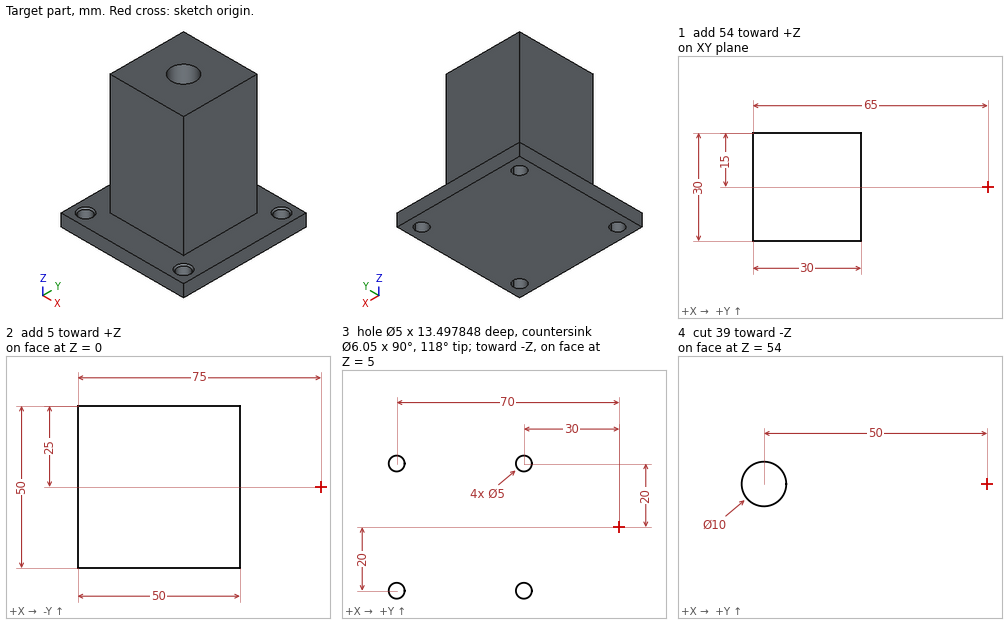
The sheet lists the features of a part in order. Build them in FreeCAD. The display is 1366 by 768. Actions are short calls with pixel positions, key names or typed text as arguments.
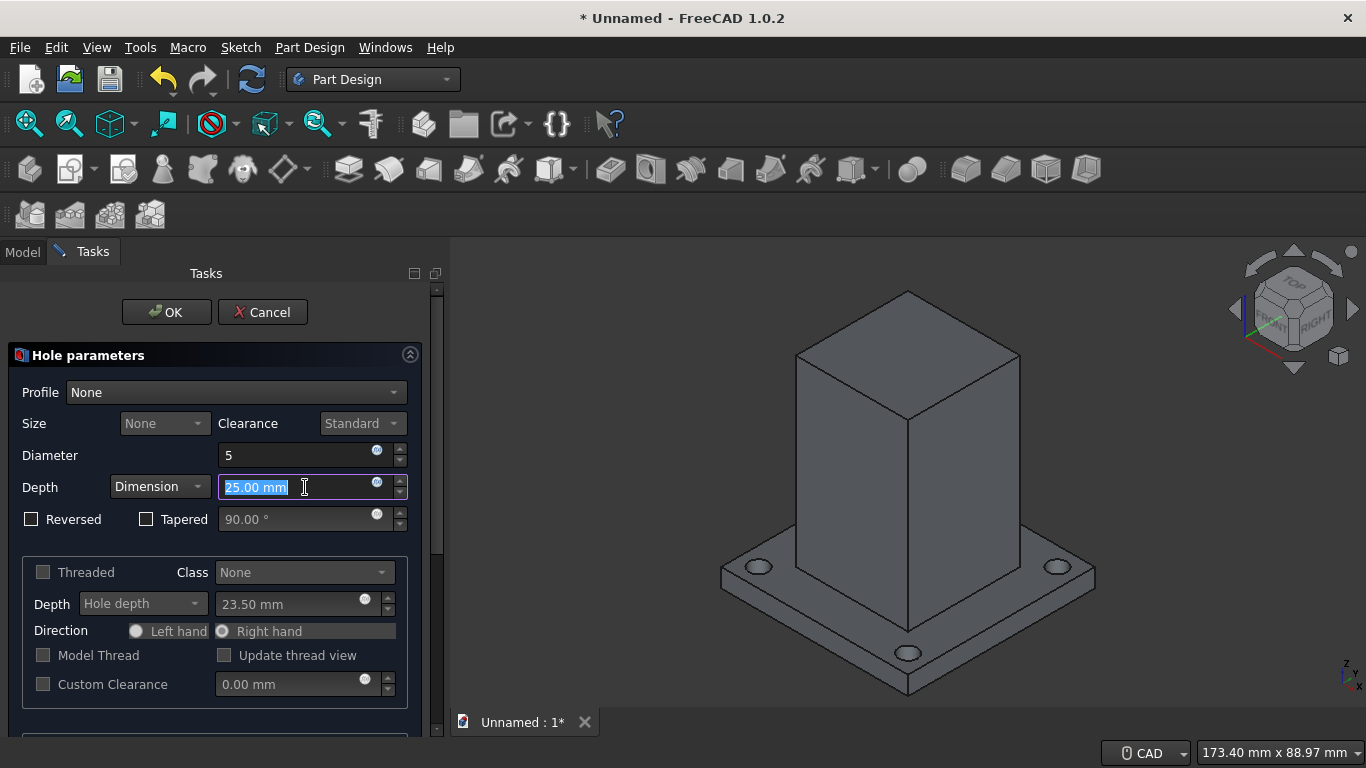
text(13.497848)
key(Tab)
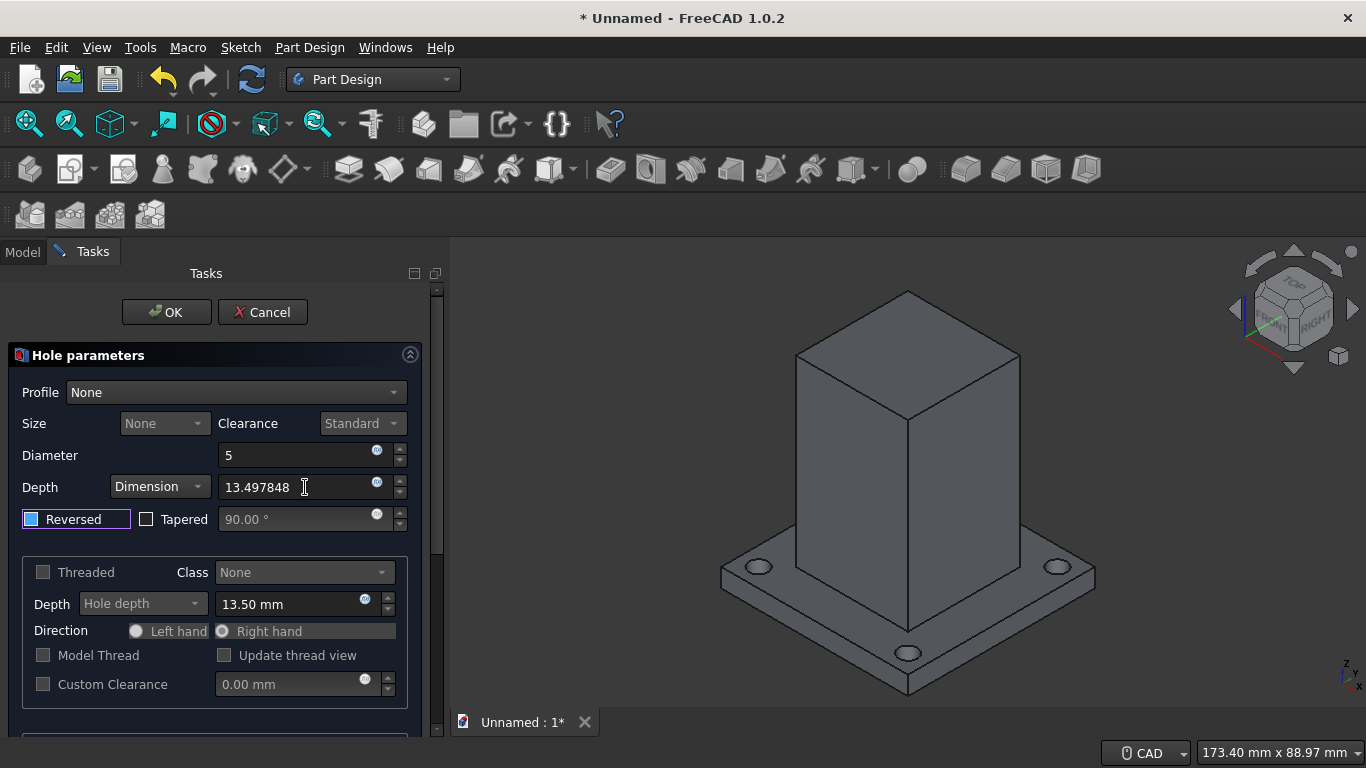
scroll(437, 510, down, 2)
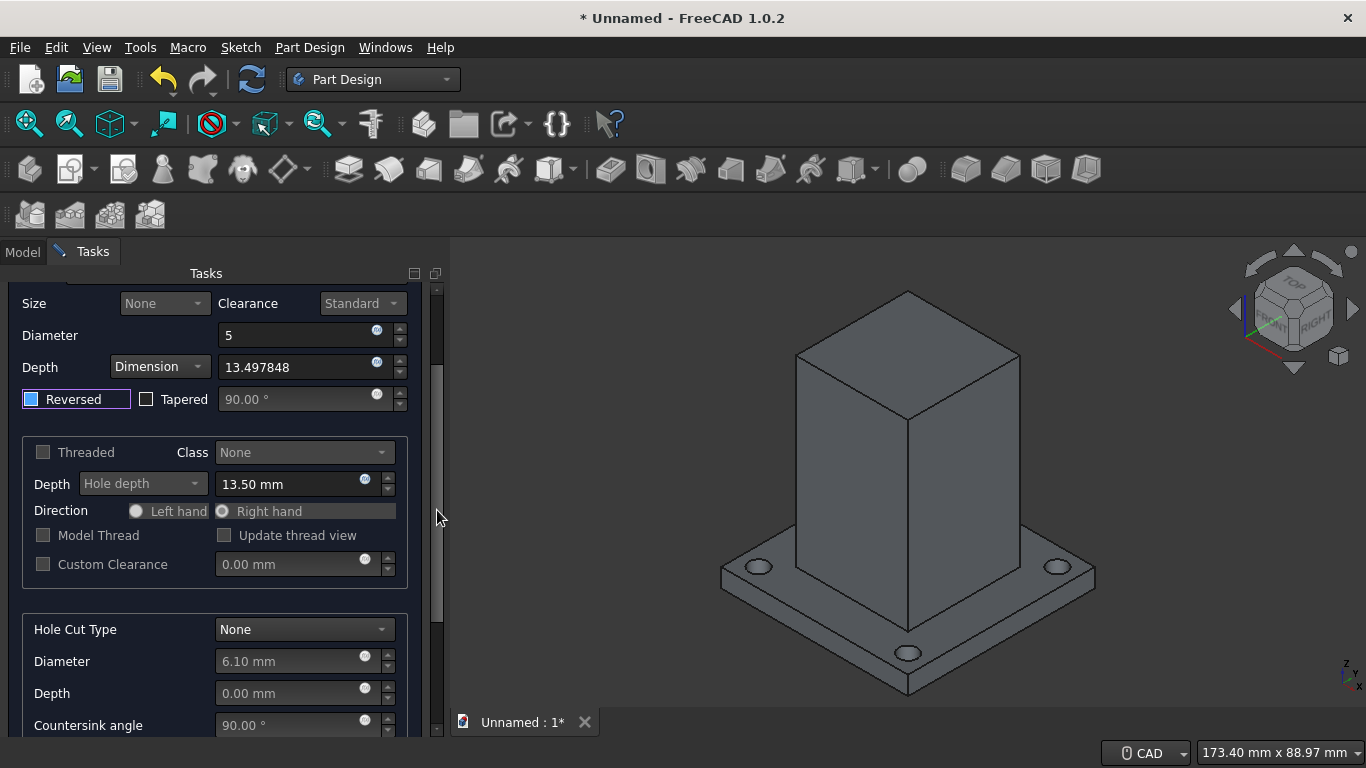
click(306, 630)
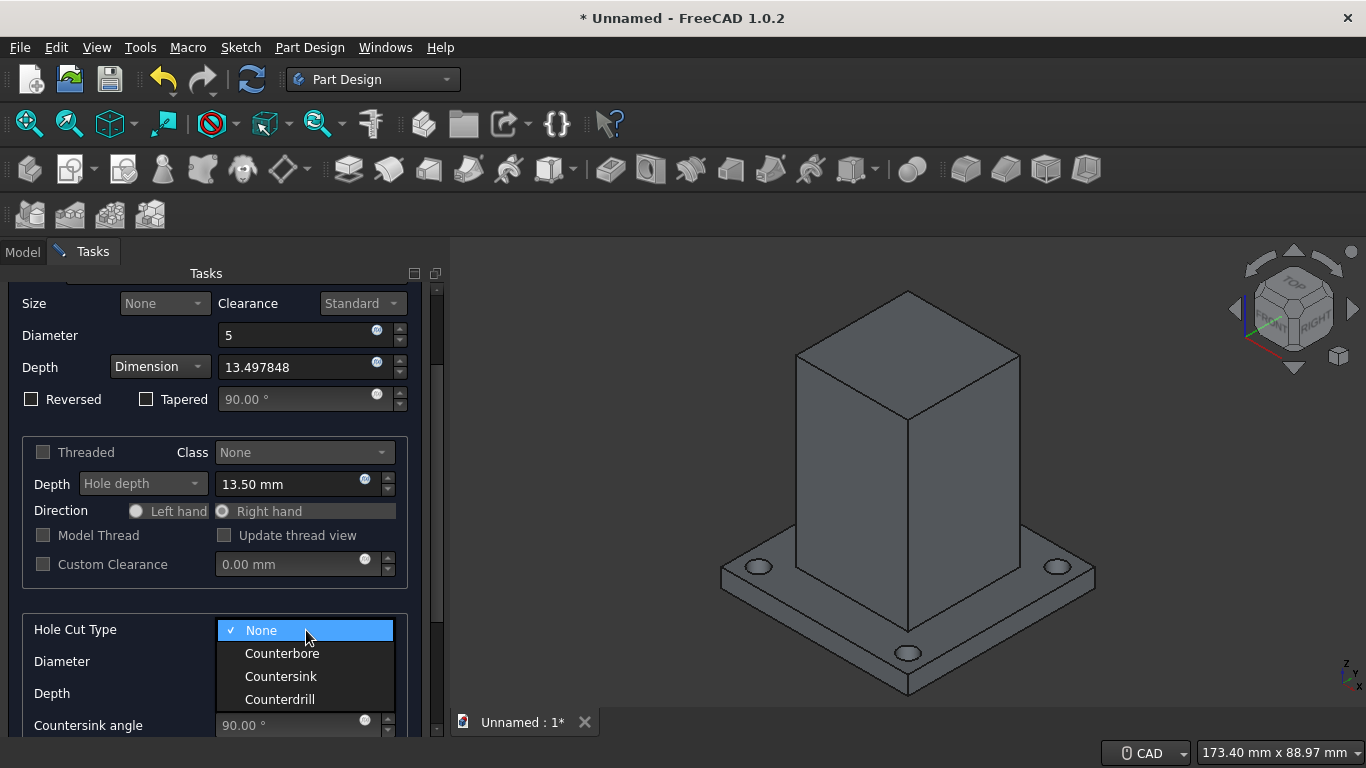
click(304, 676)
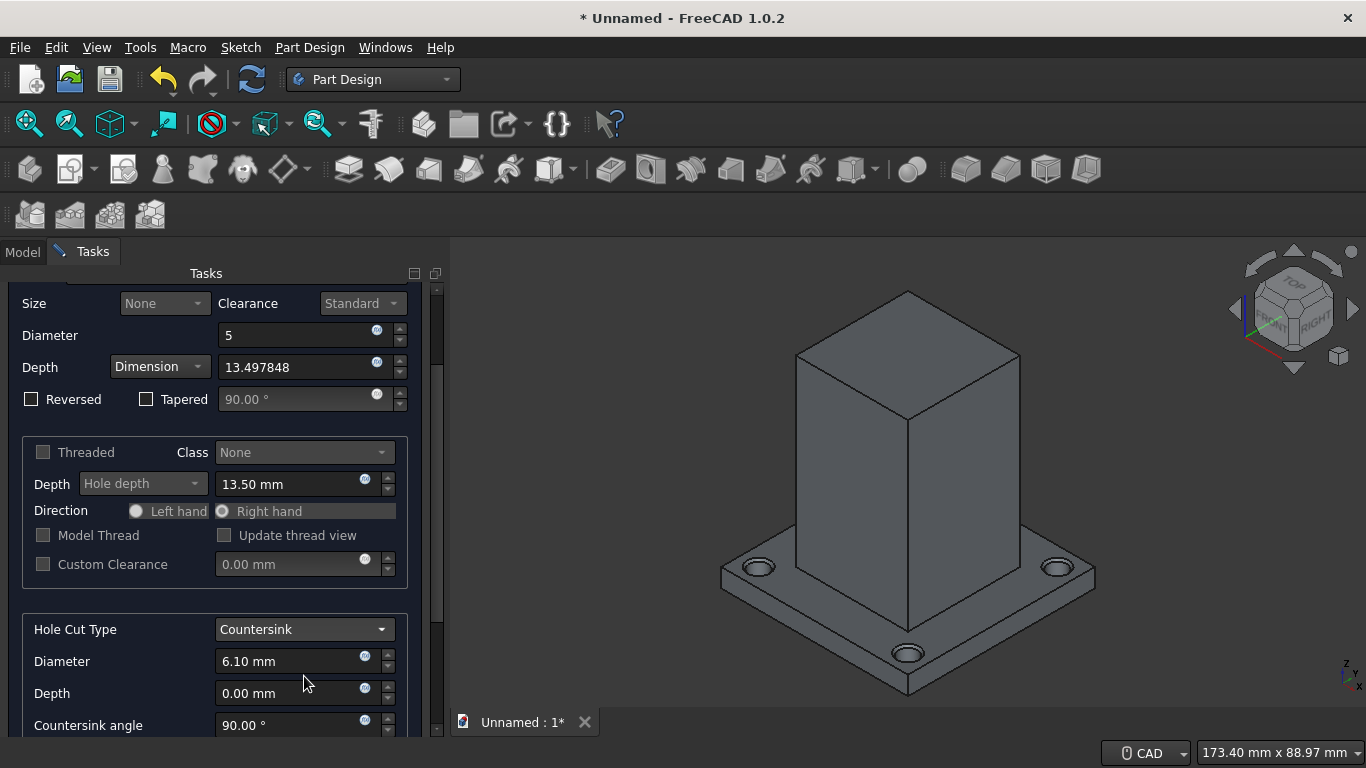
triple_click(298, 661)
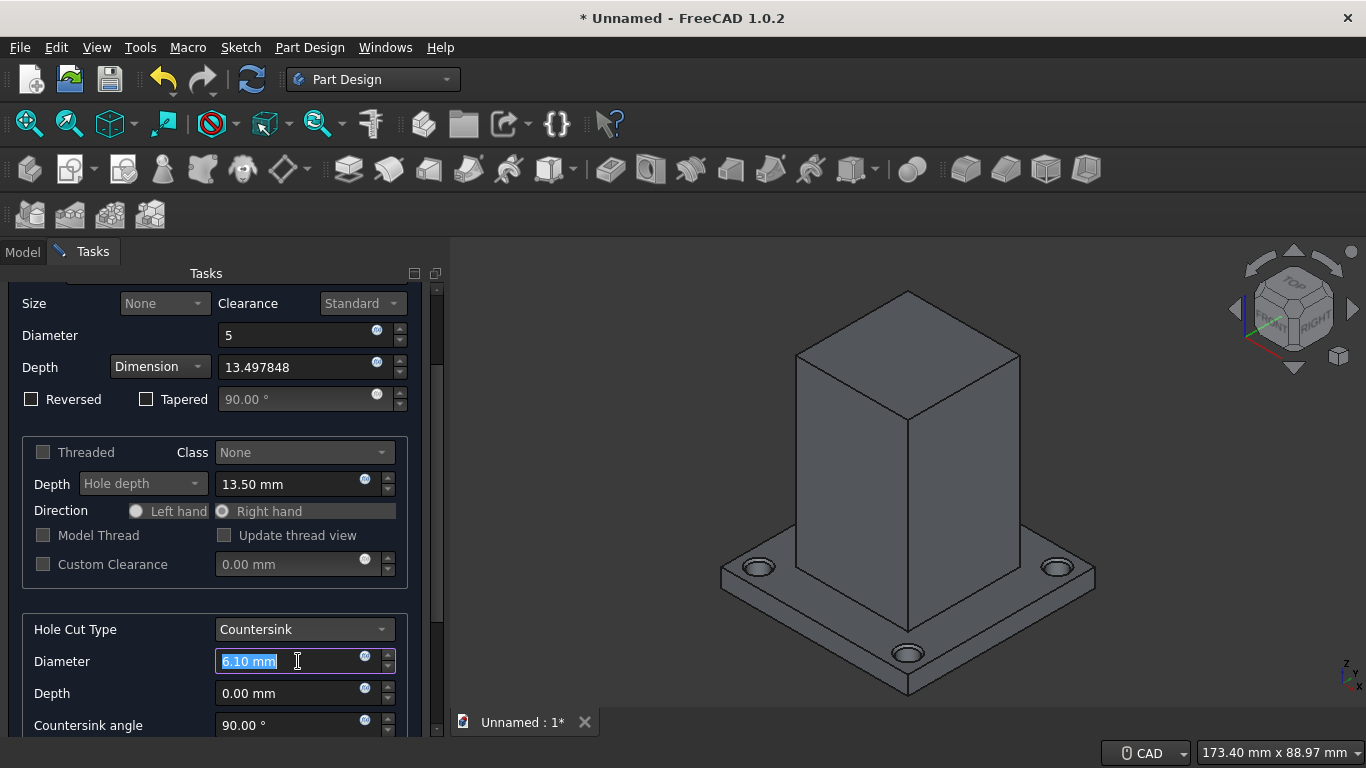
text(6.05)
key(Tab)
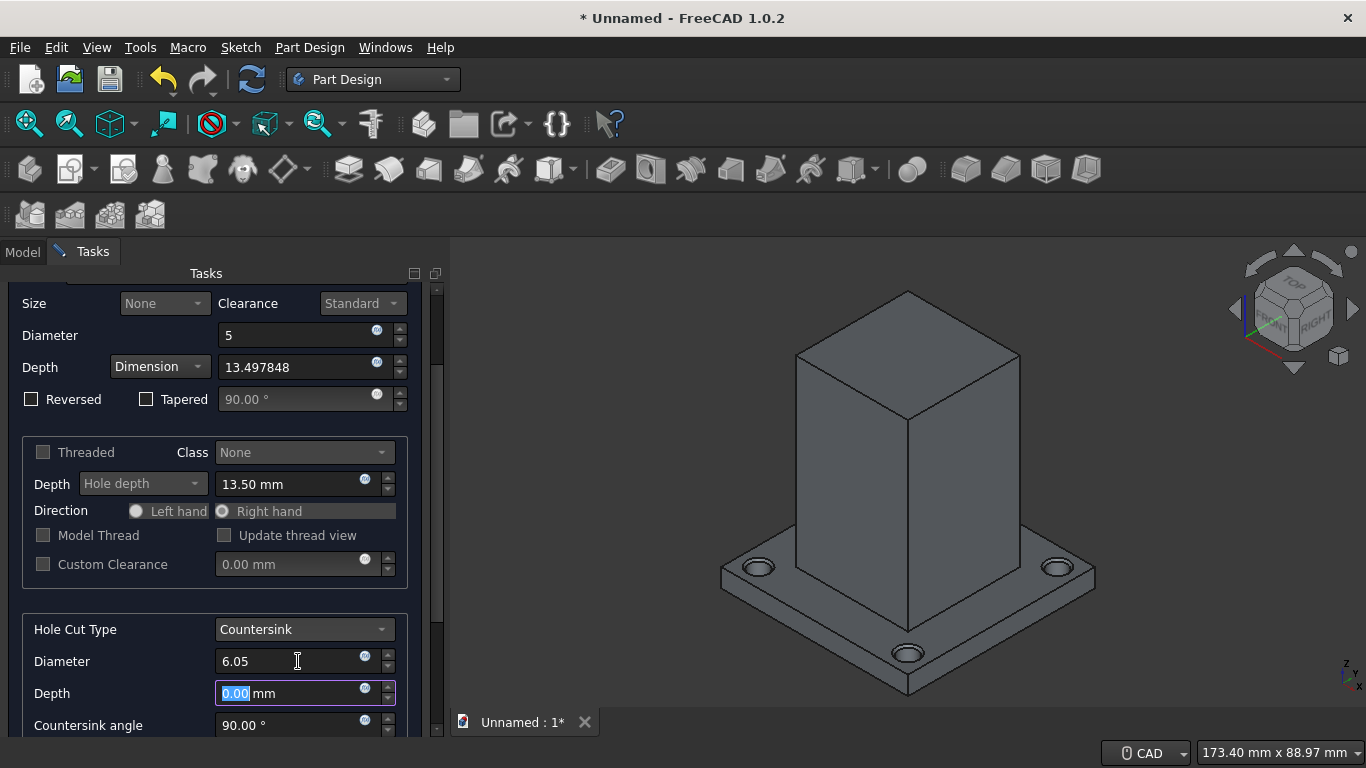
scroll(437, 510, up, 3)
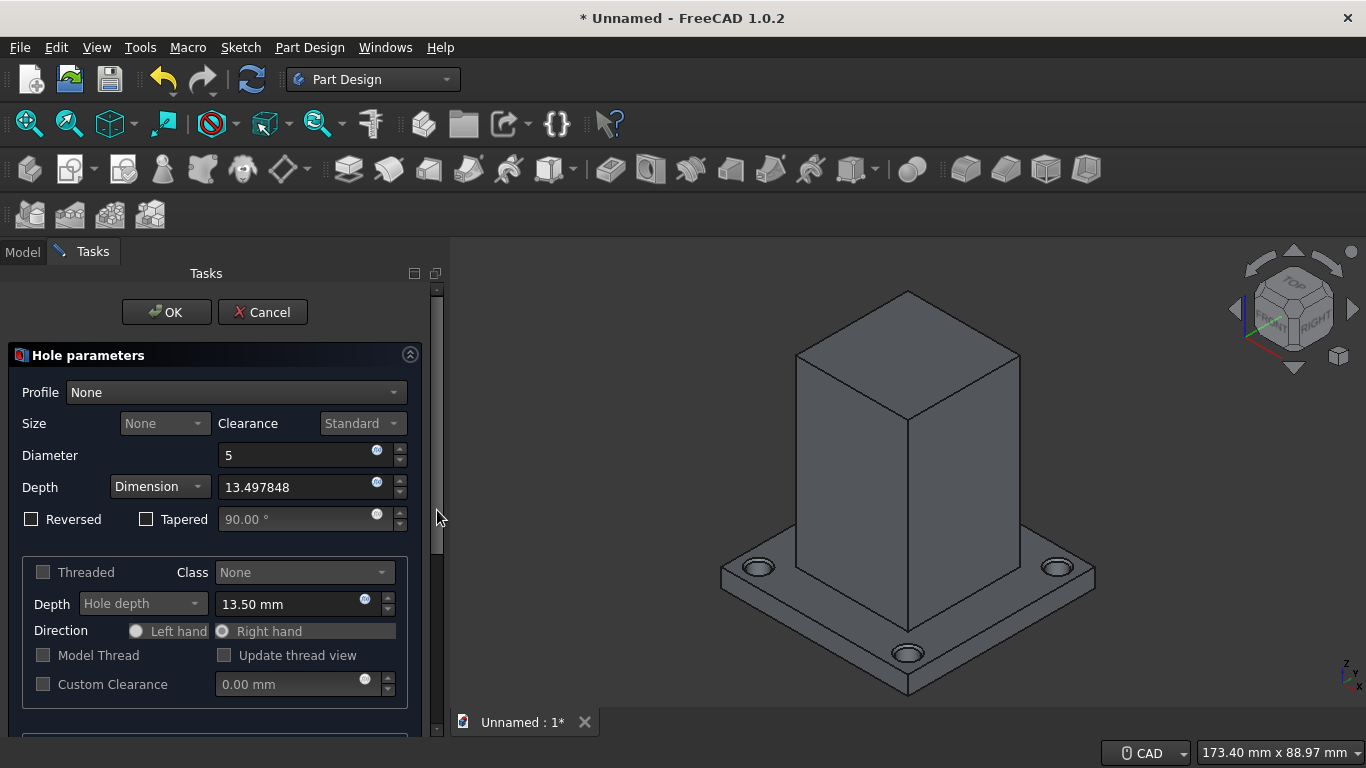
click(167, 312)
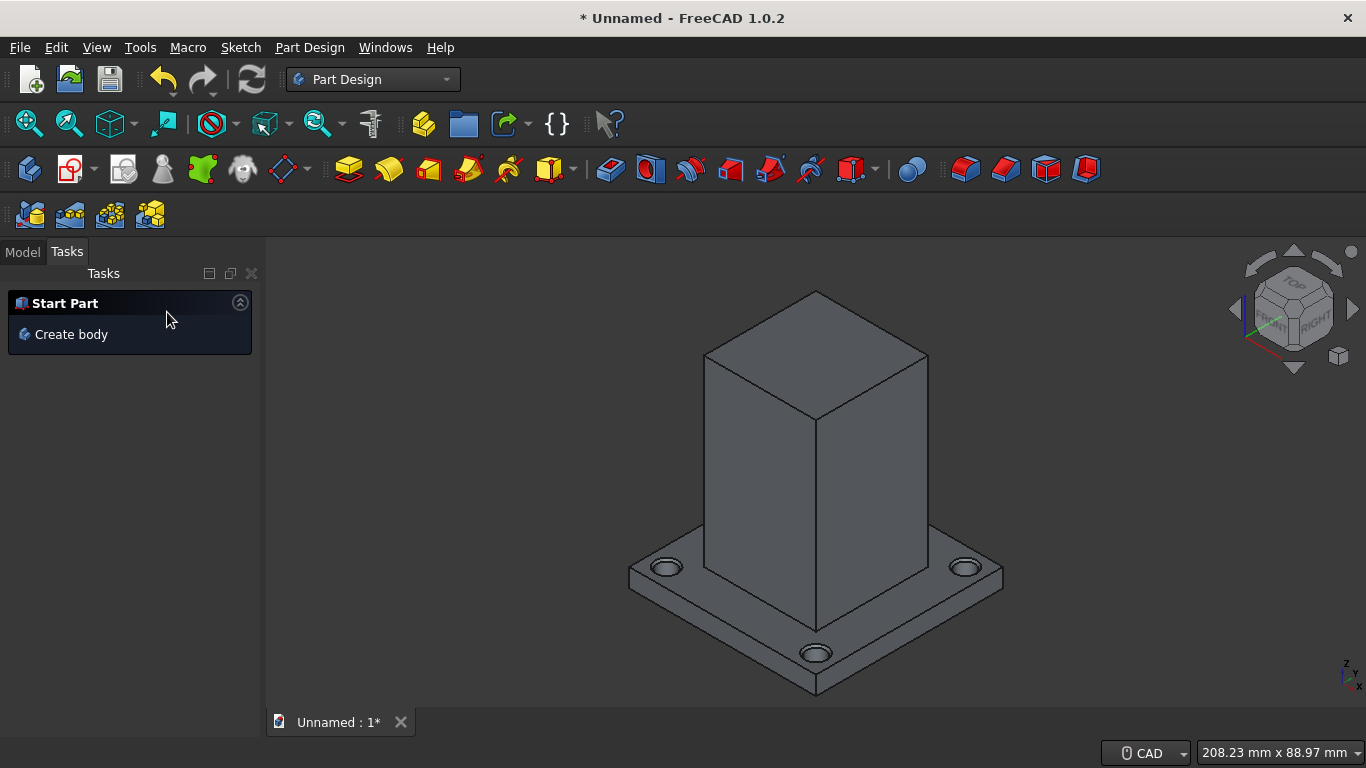
click(816, 355)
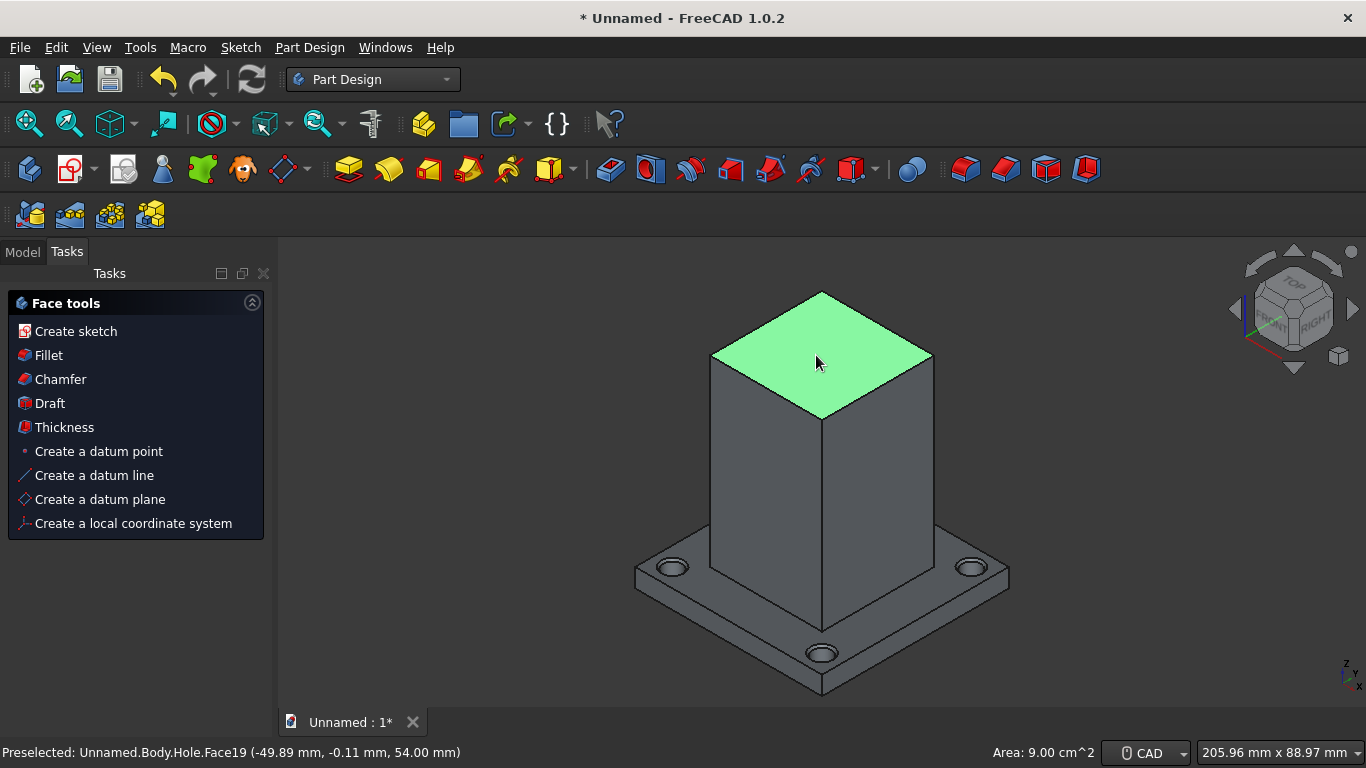
click(70, 170)